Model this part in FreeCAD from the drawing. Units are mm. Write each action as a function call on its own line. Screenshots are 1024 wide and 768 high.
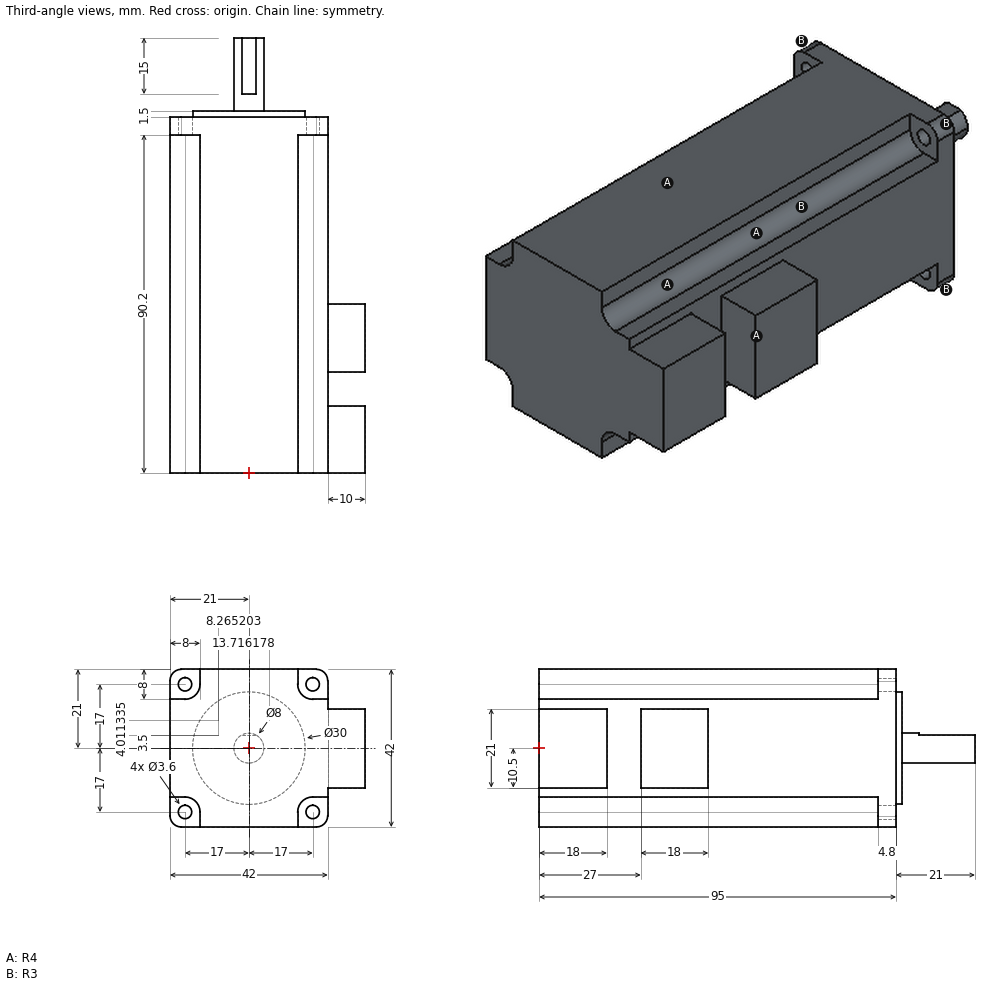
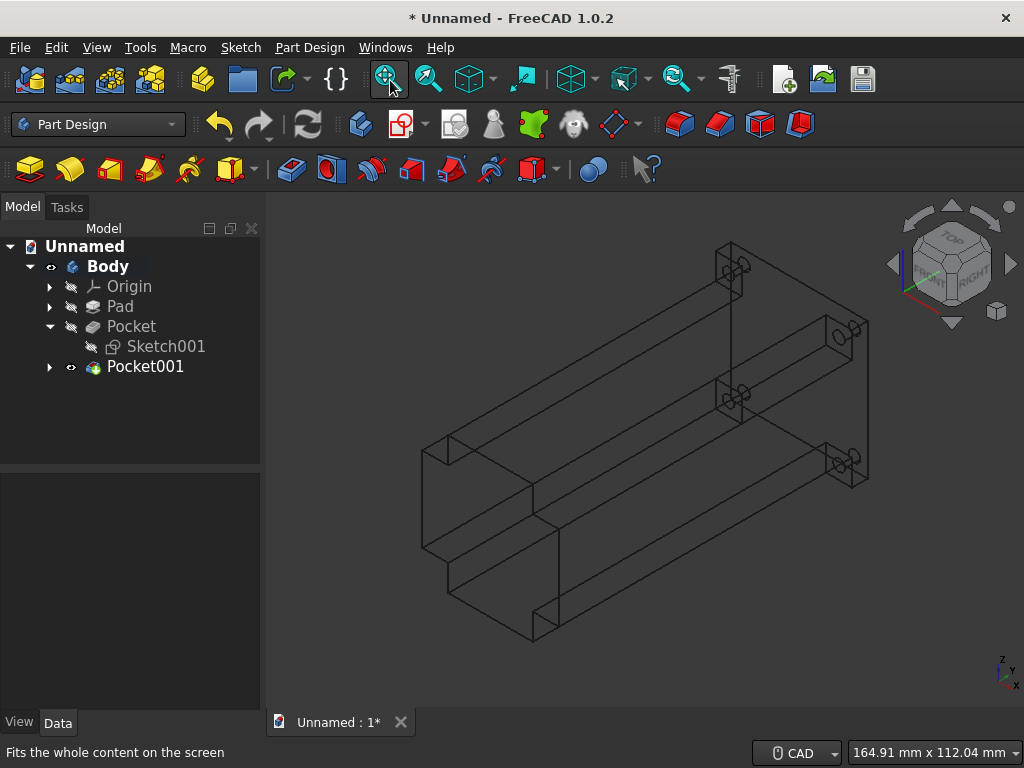
click(595, 380)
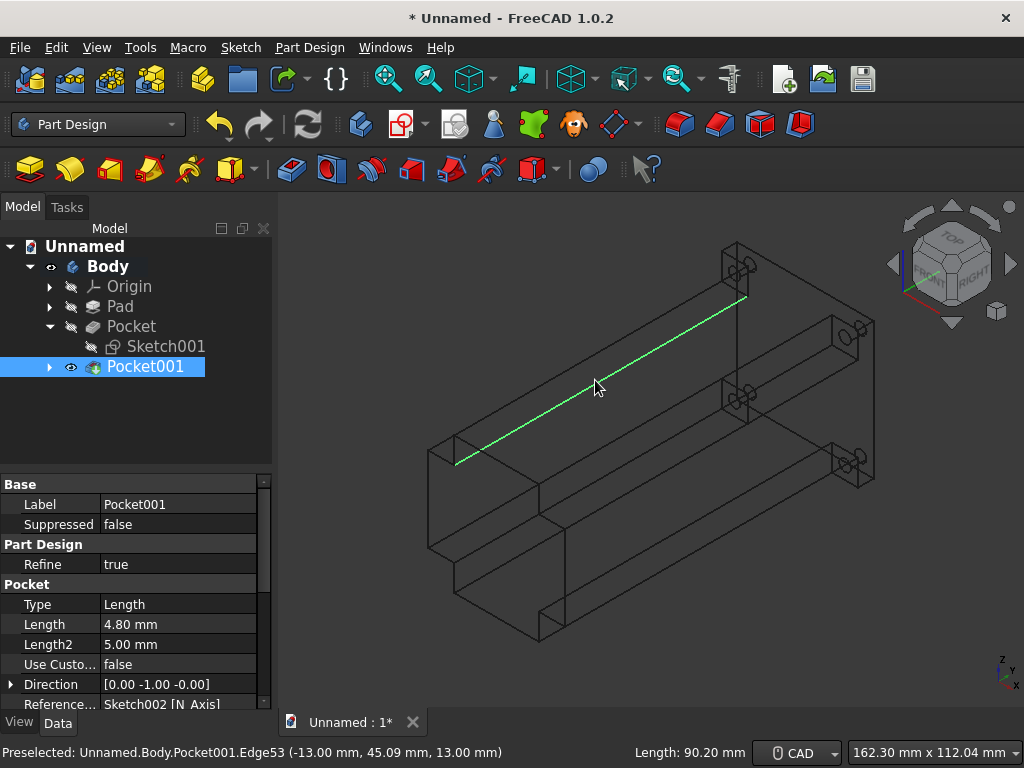
click(685, 429, ctrl)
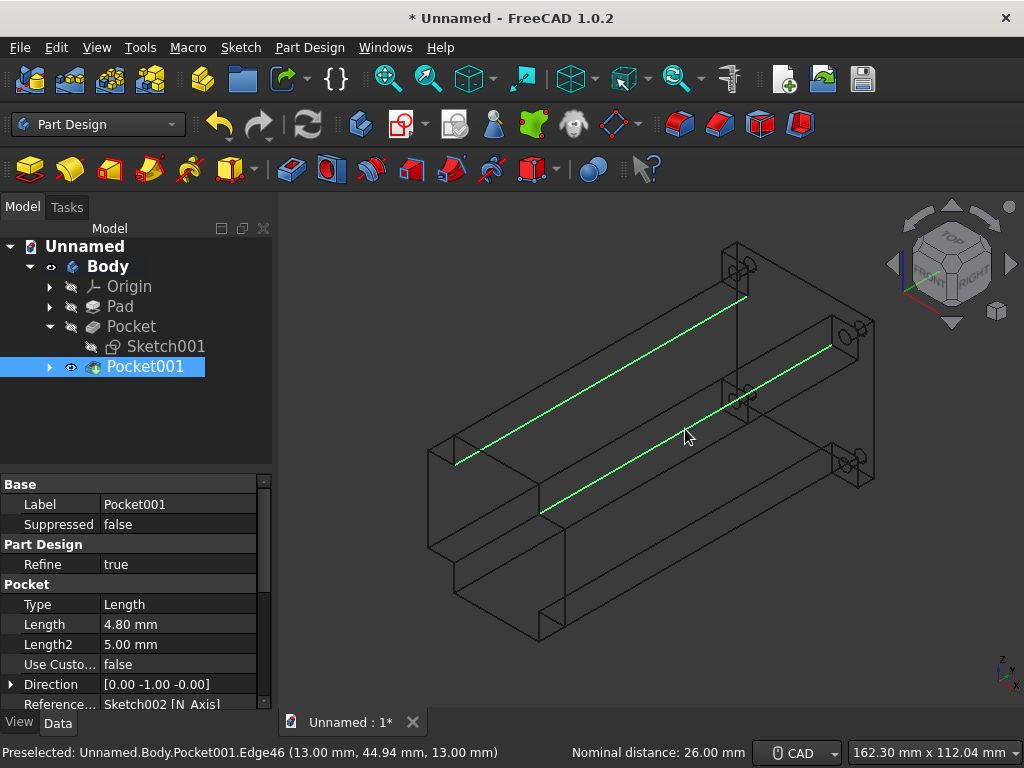
click(513, 528, ctrl)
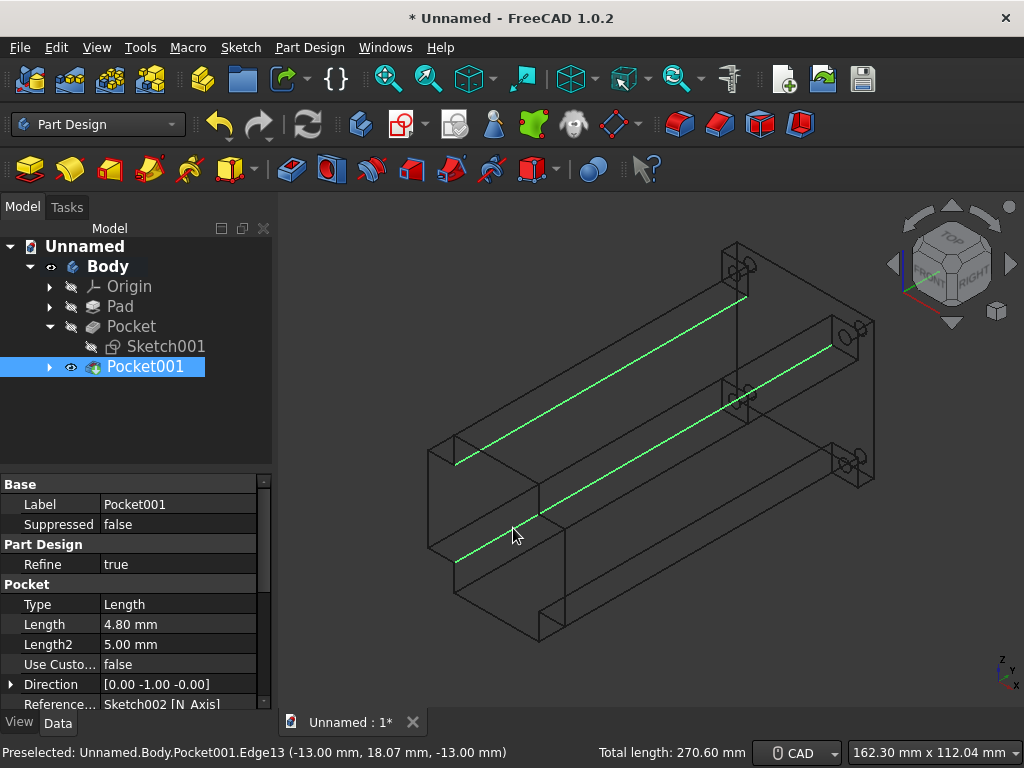
click(685, 526, ctrl)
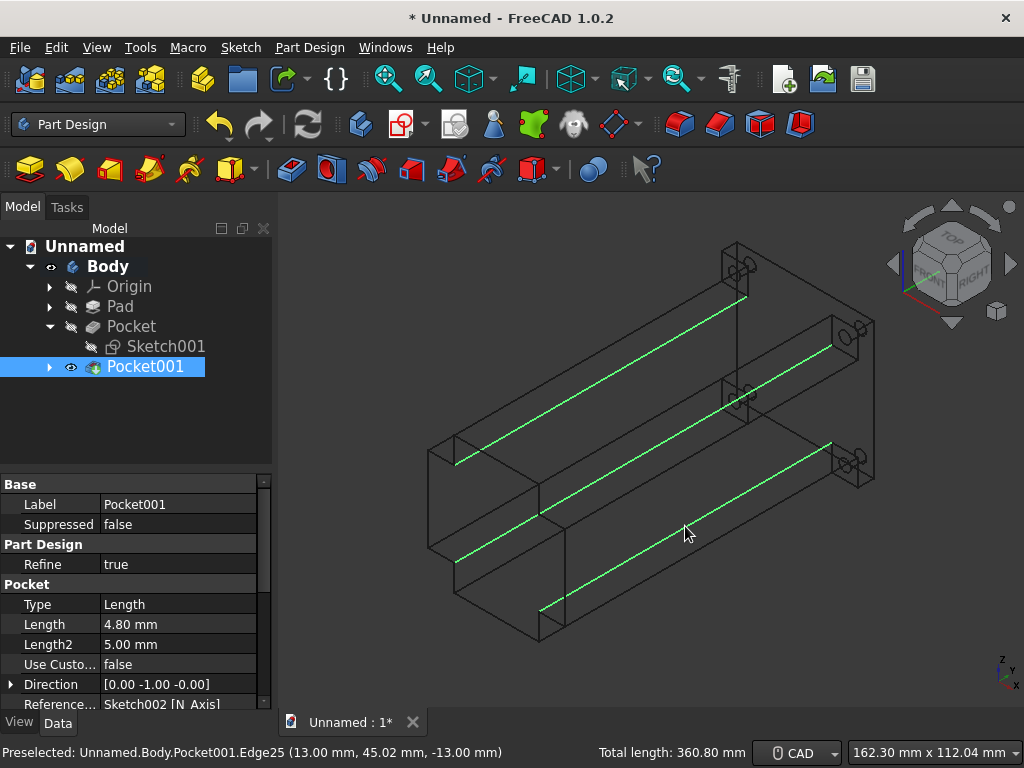
key(v)
key(1)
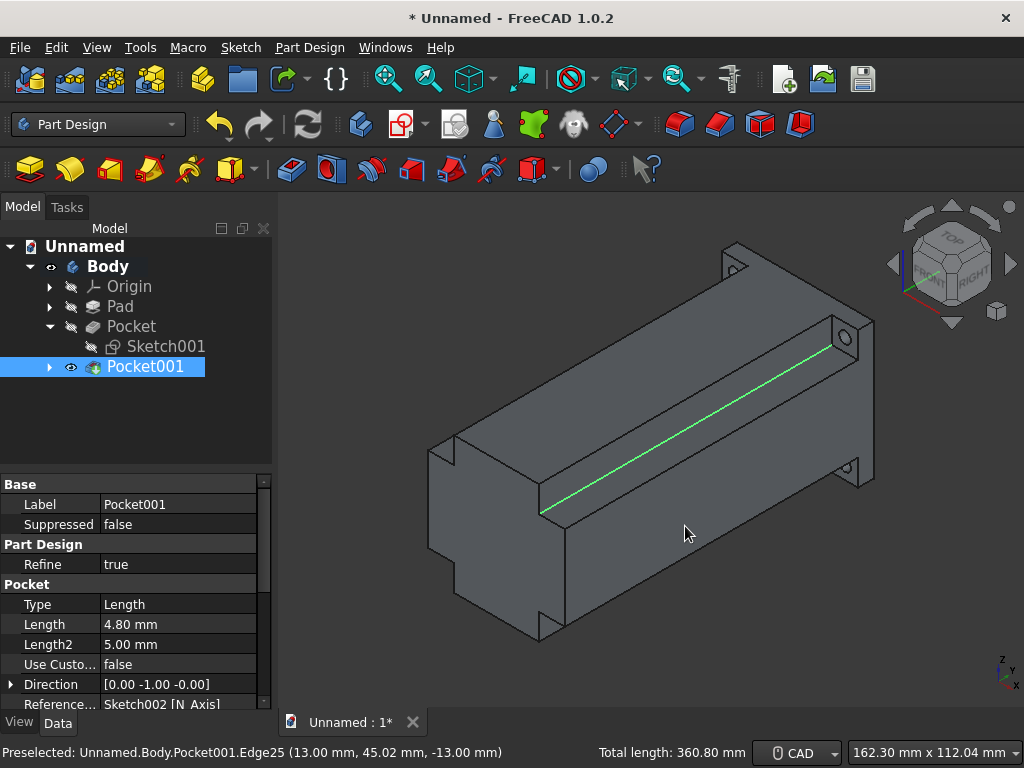
click(680, 124)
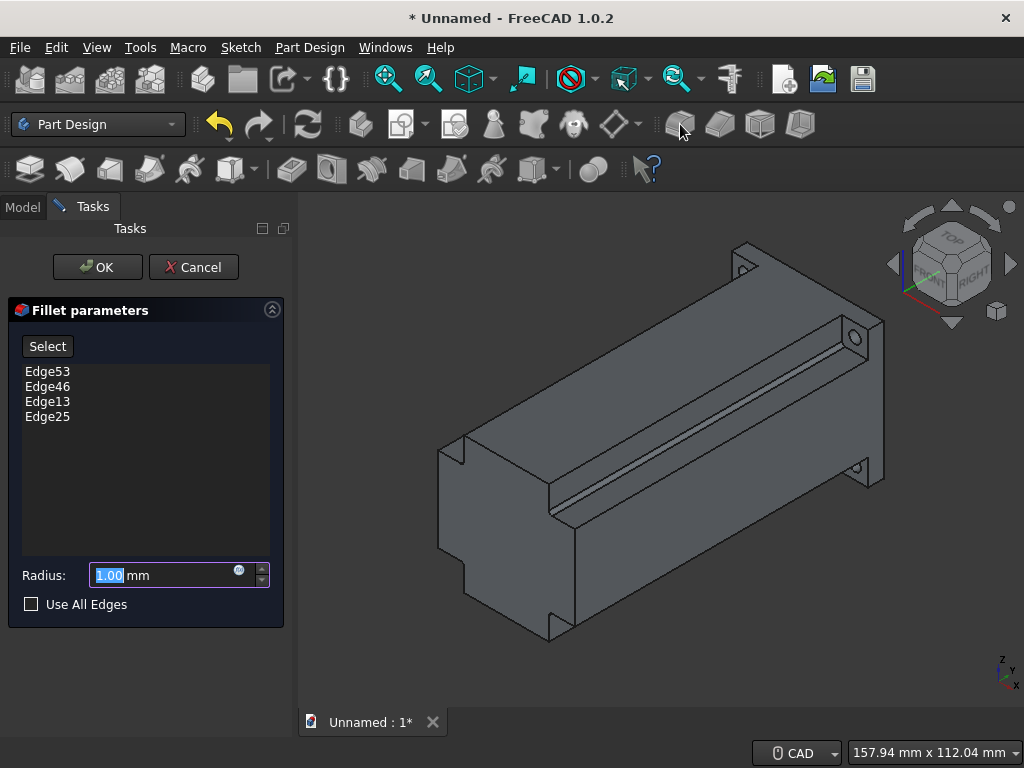
text(4)
key(Tab)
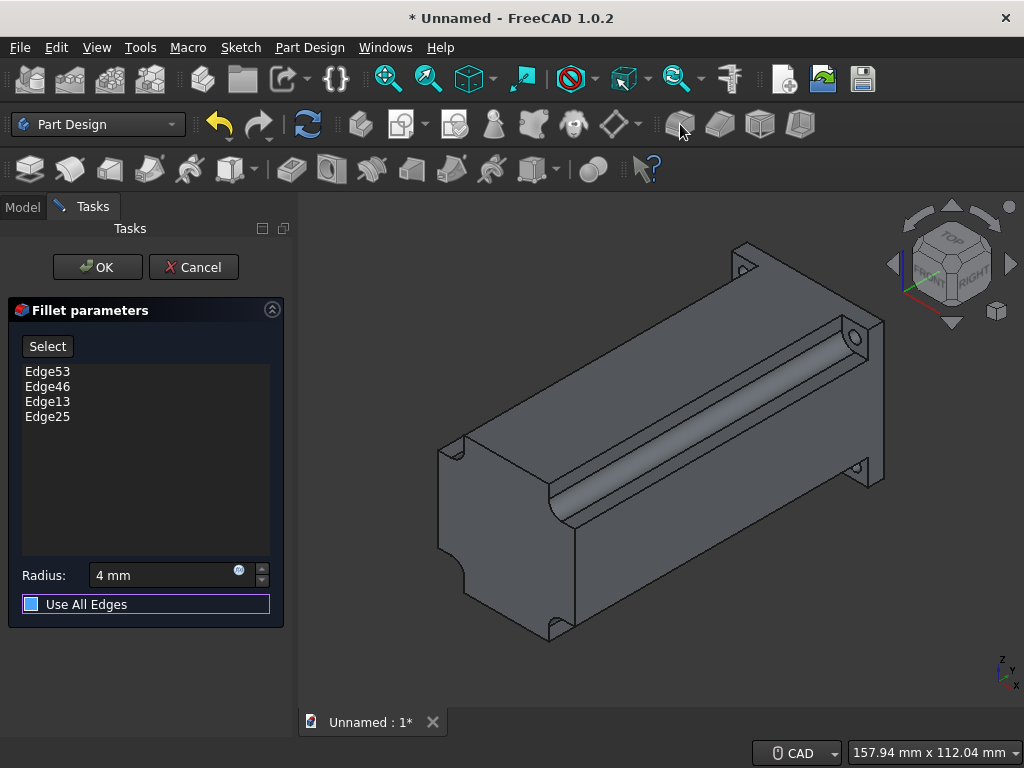
click(98, 267)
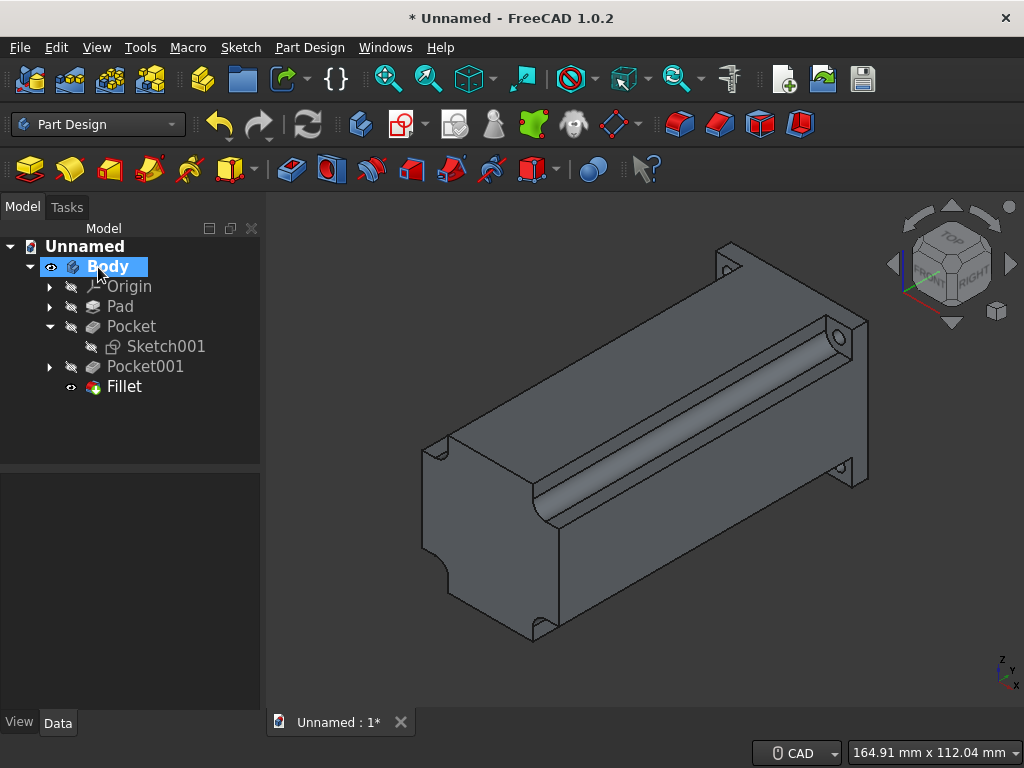
key(4)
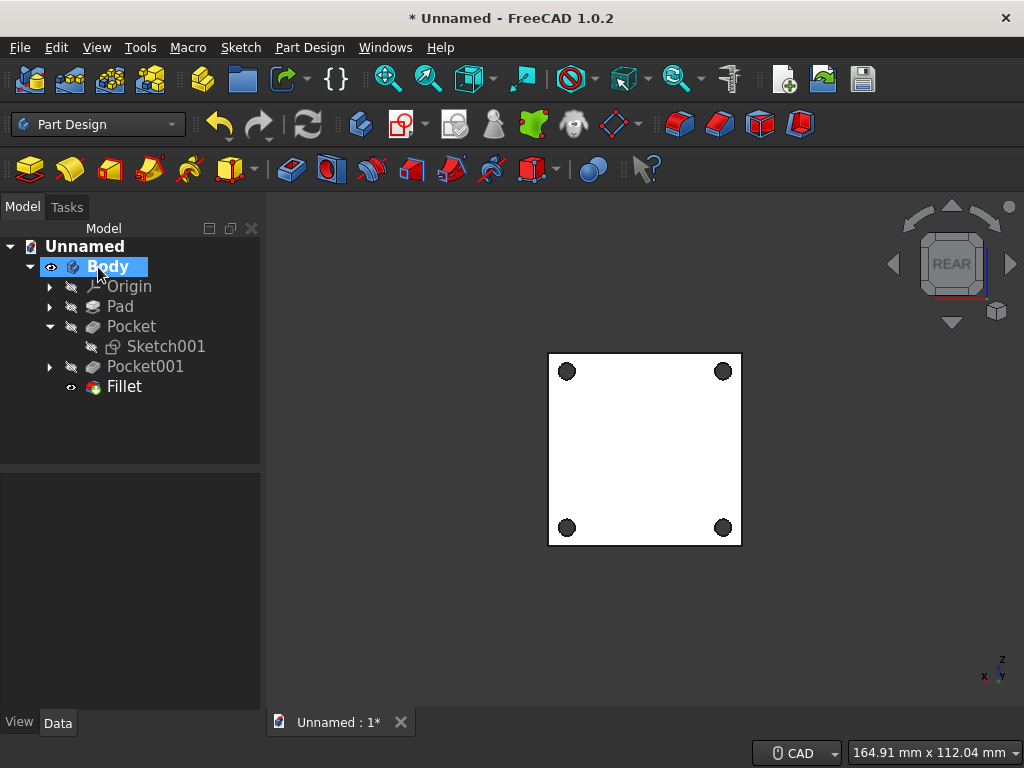
click(390, 80)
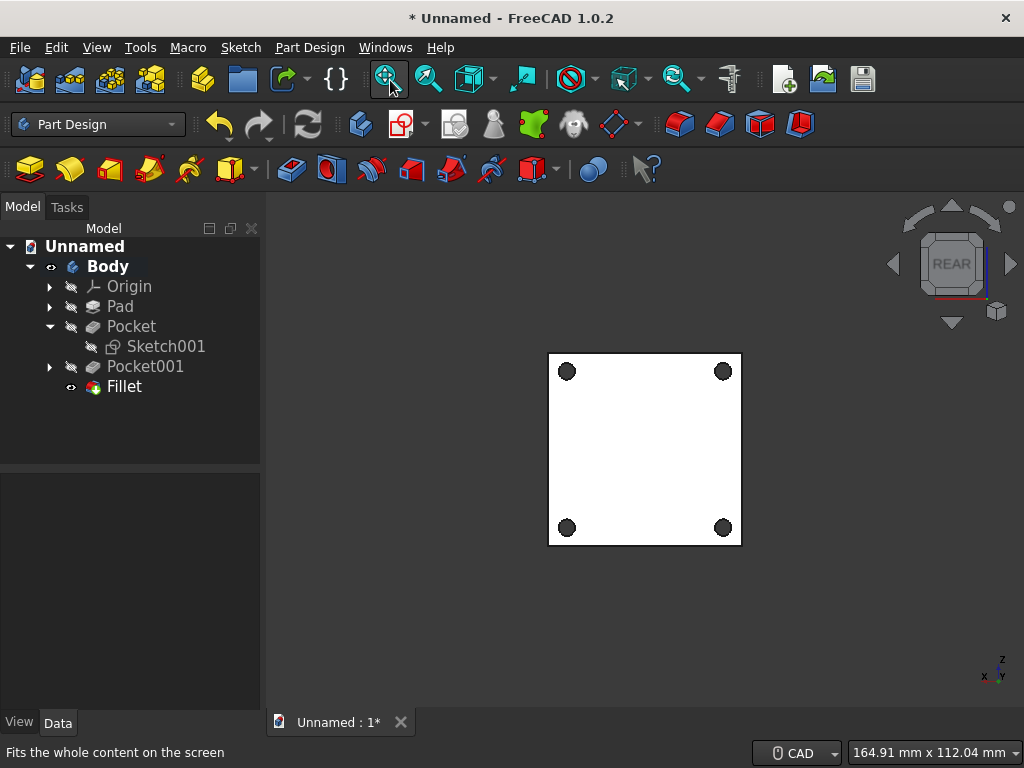
click(645, 449)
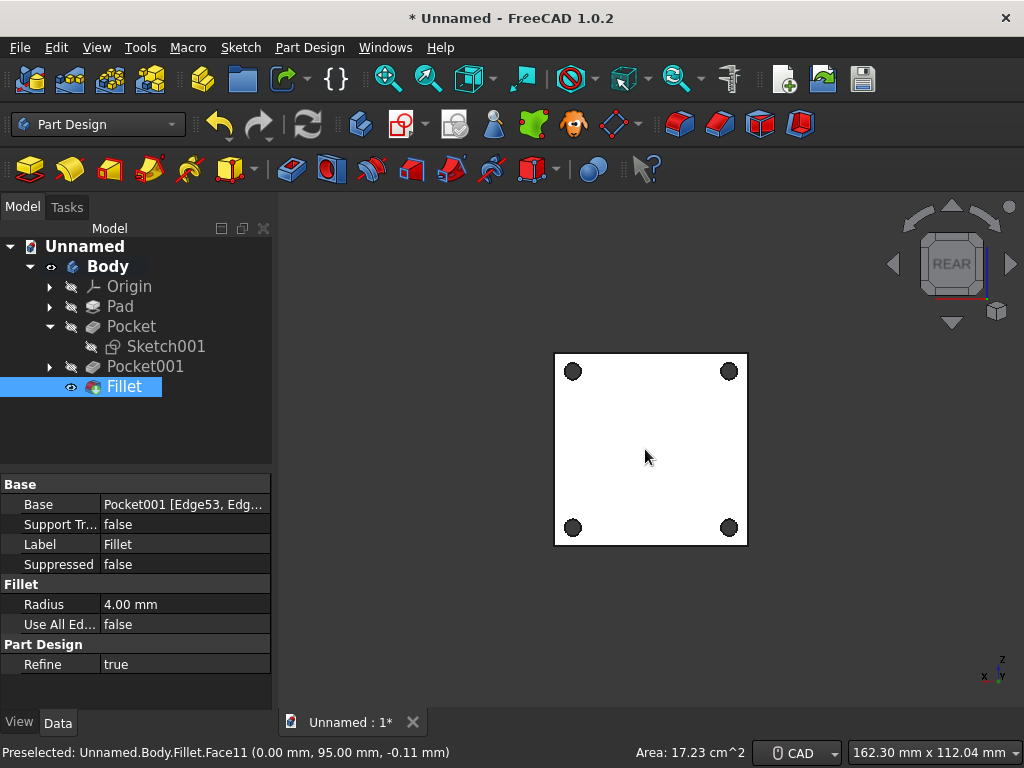
click(402, 124)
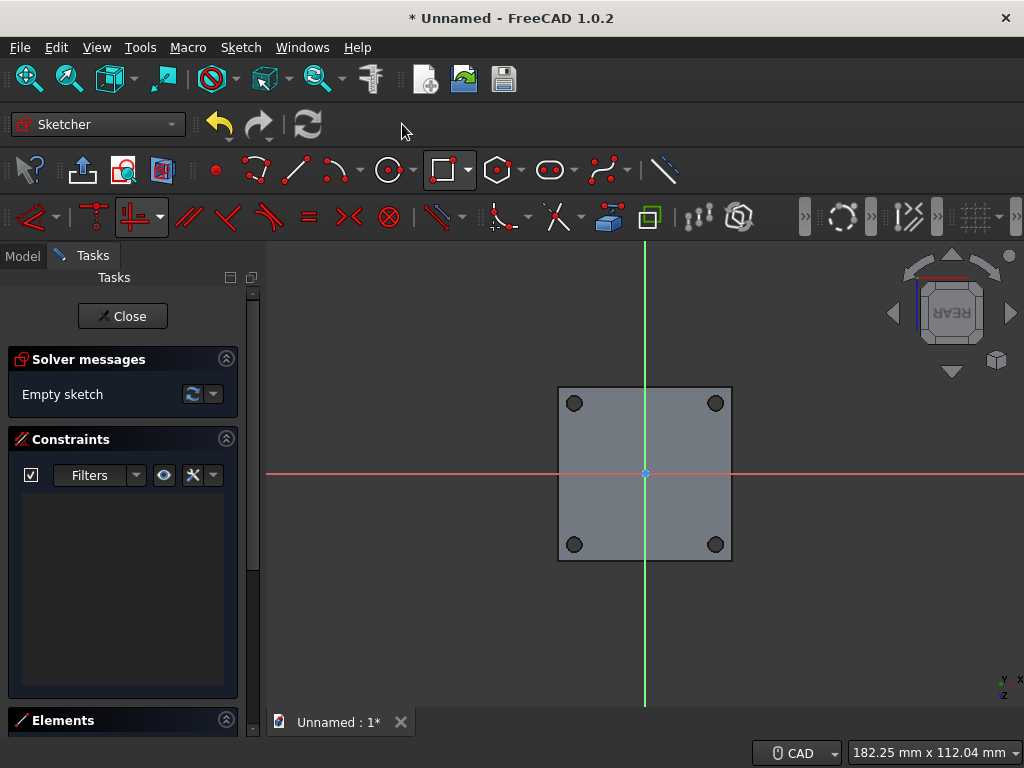
scroll(701, 474, up, 4)